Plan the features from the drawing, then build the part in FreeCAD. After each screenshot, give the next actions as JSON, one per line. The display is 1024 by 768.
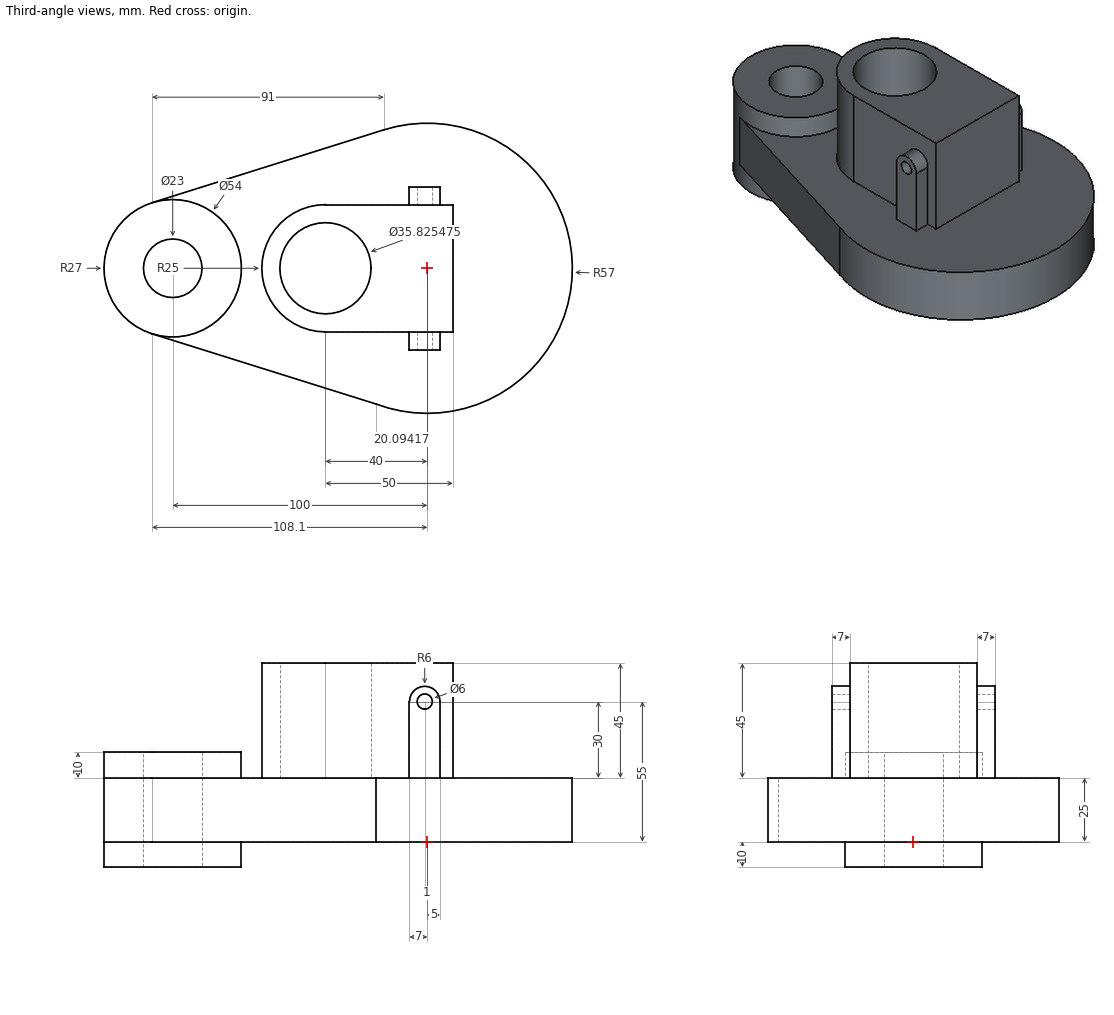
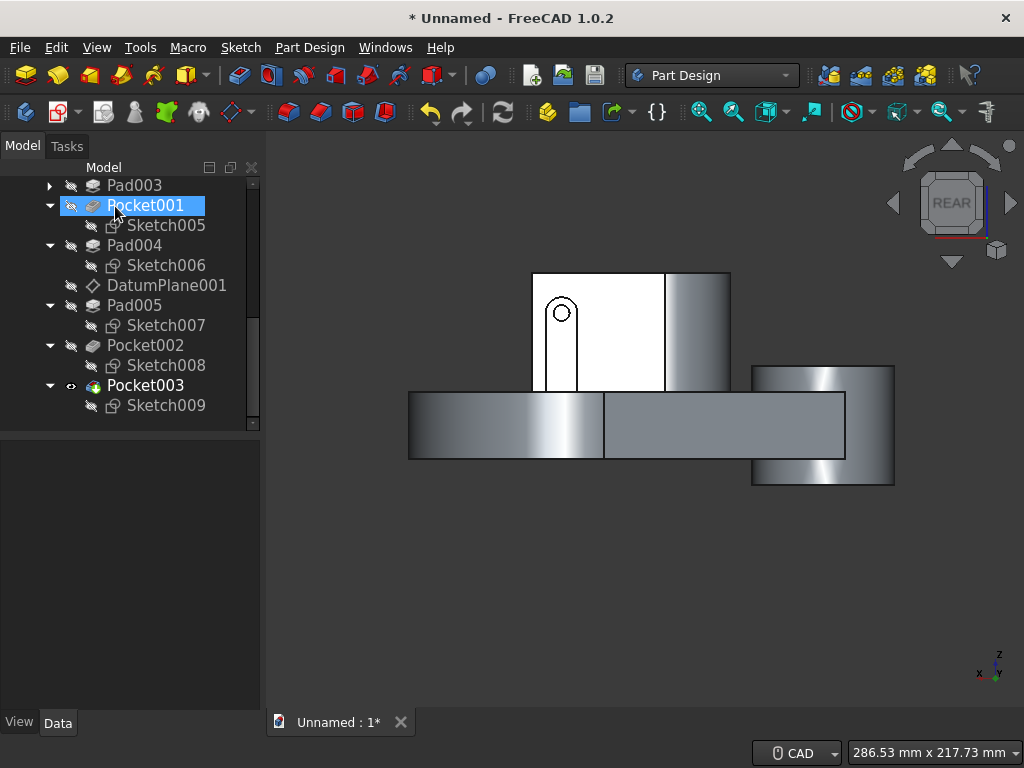
{"action": "key", "text": "0"}